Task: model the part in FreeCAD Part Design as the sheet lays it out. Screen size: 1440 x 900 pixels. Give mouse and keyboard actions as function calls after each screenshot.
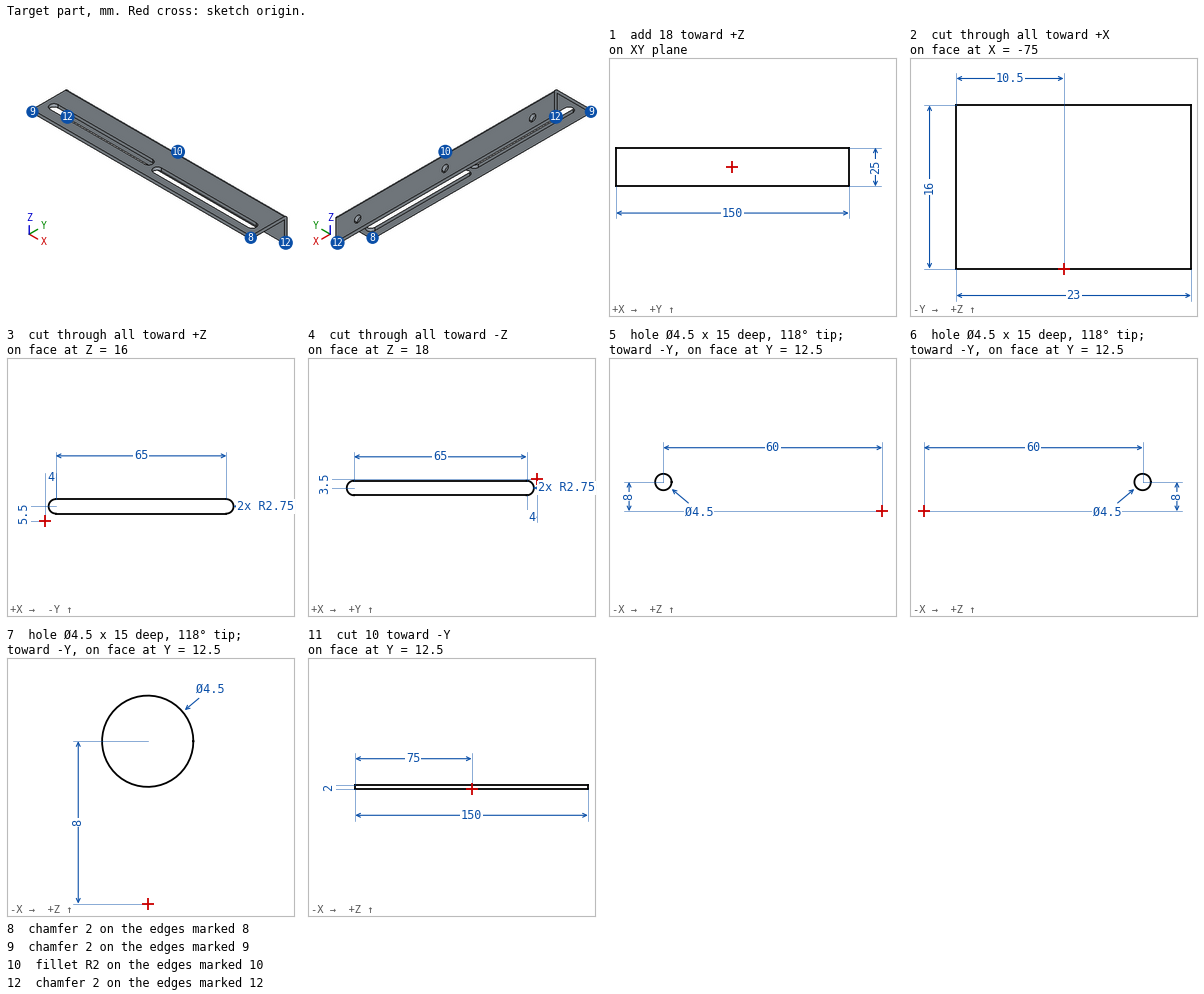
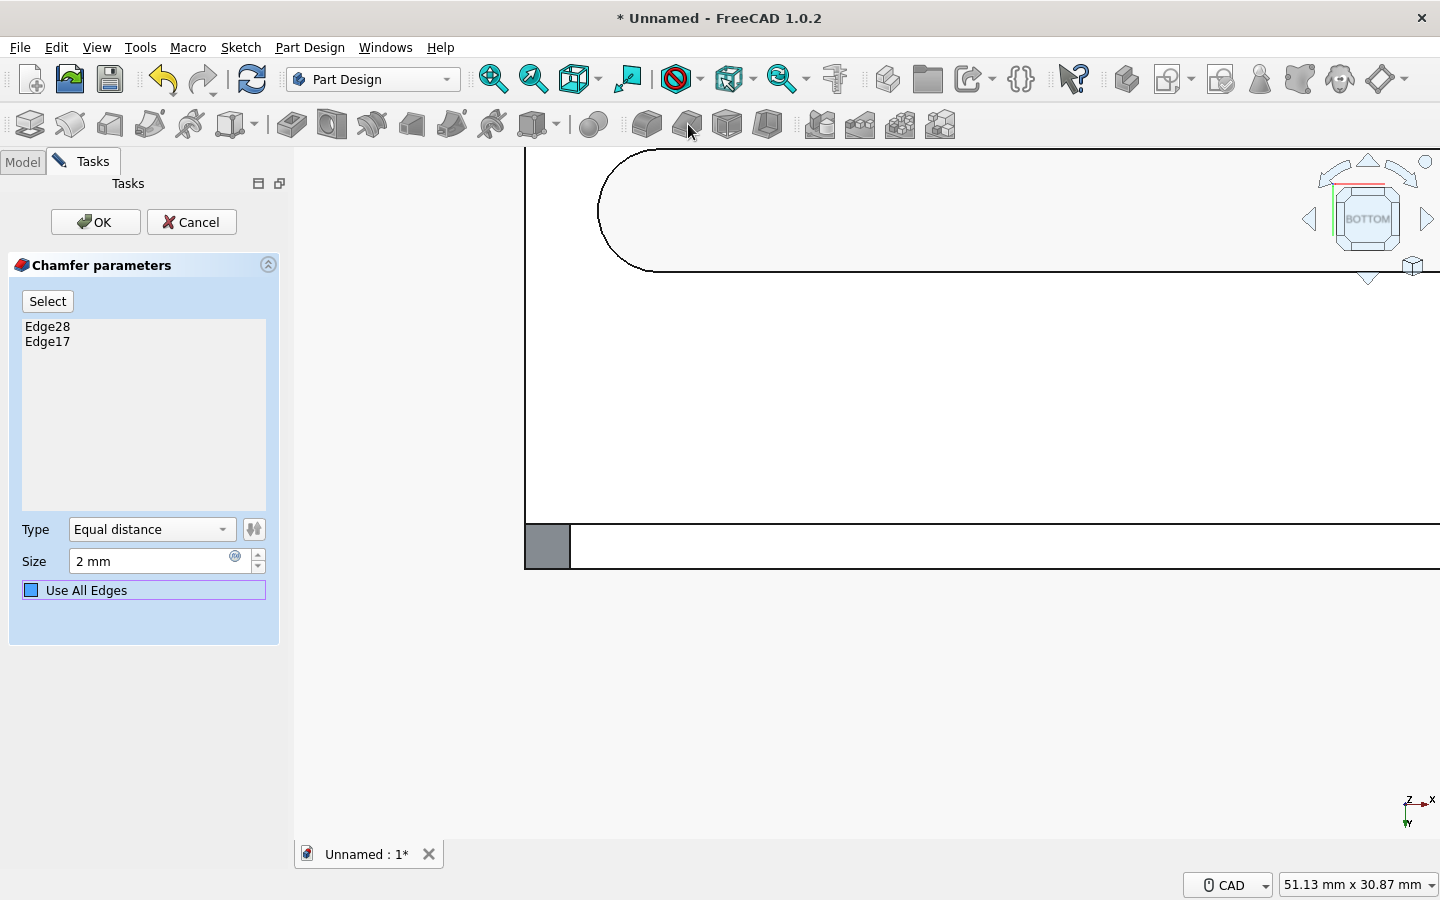
click(96, 222)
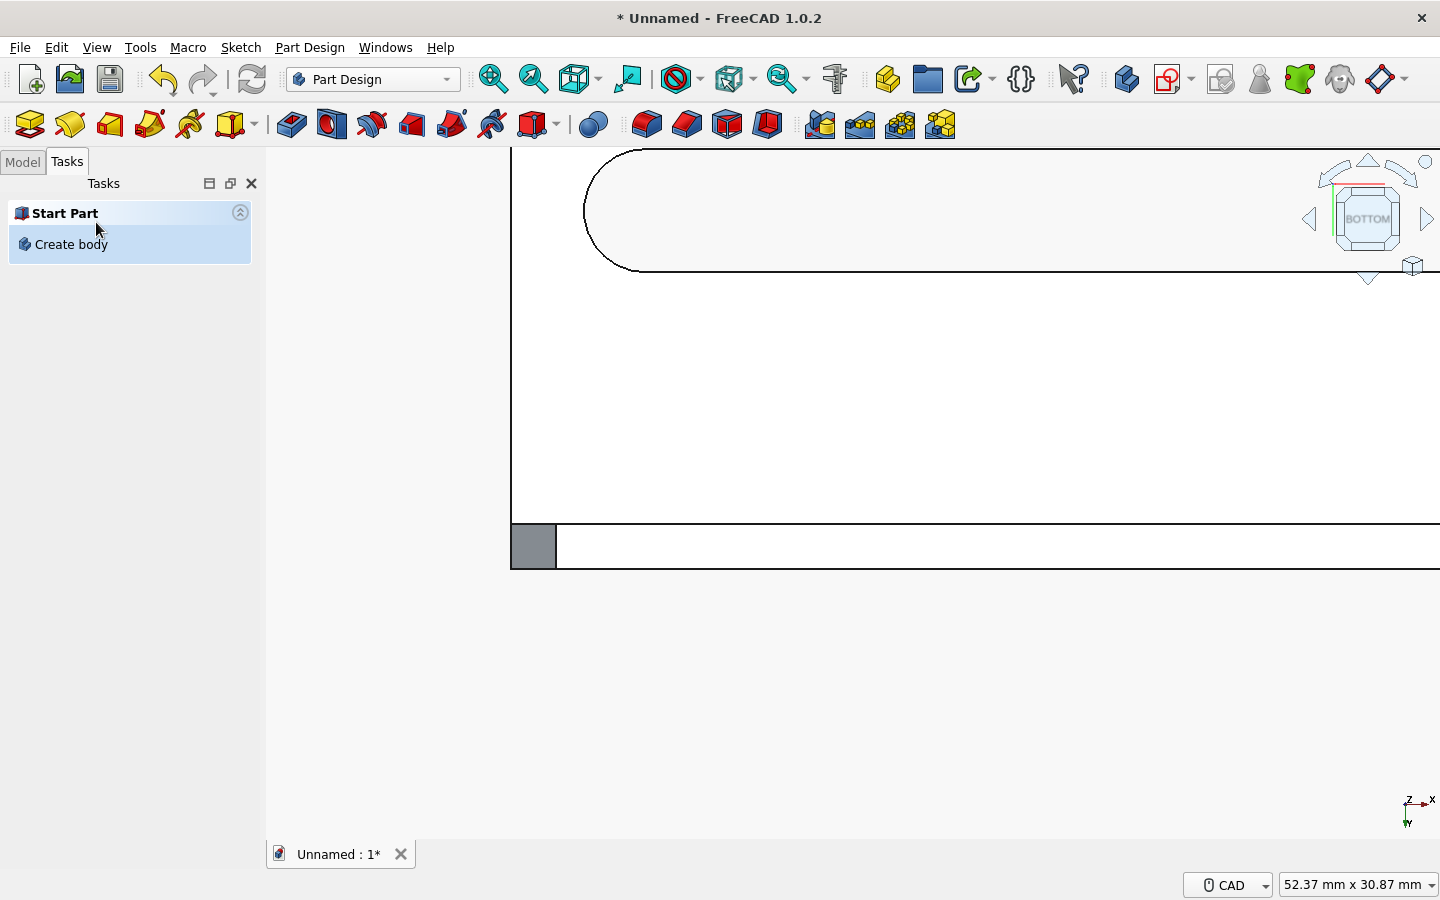
key(0)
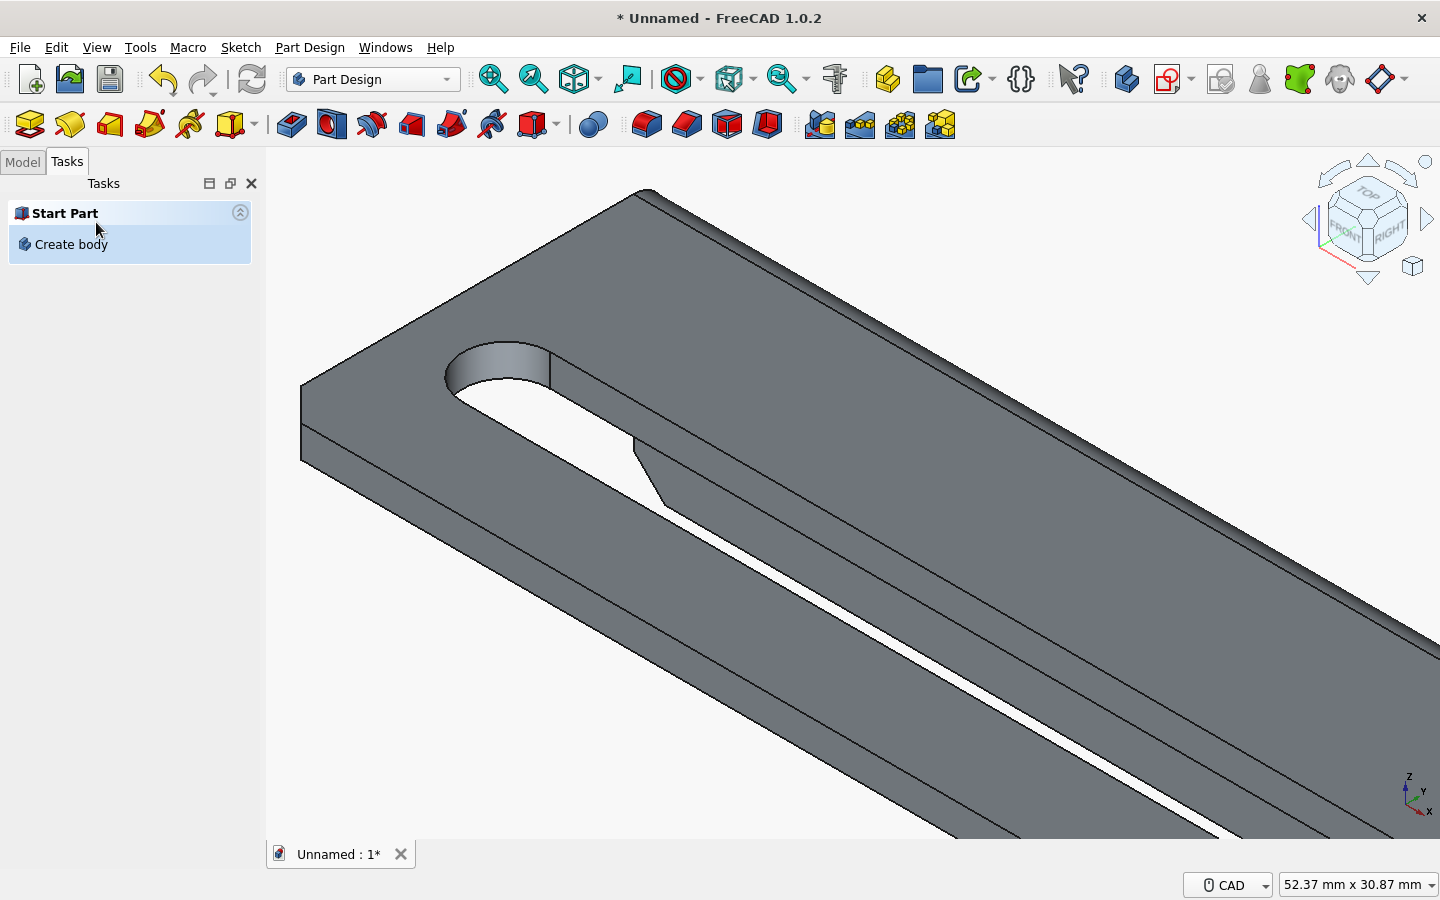
click(494, 80)